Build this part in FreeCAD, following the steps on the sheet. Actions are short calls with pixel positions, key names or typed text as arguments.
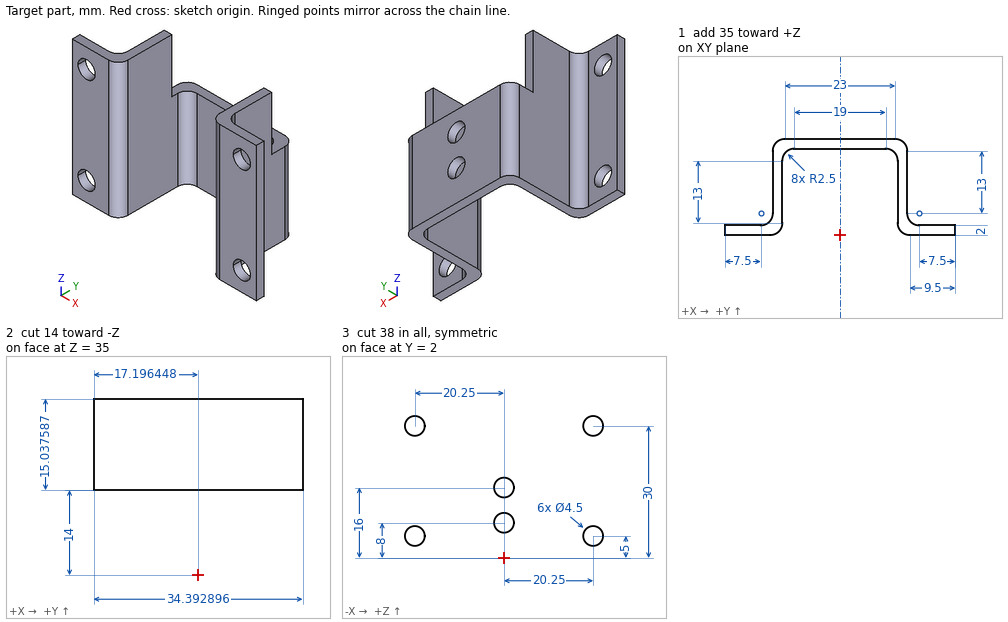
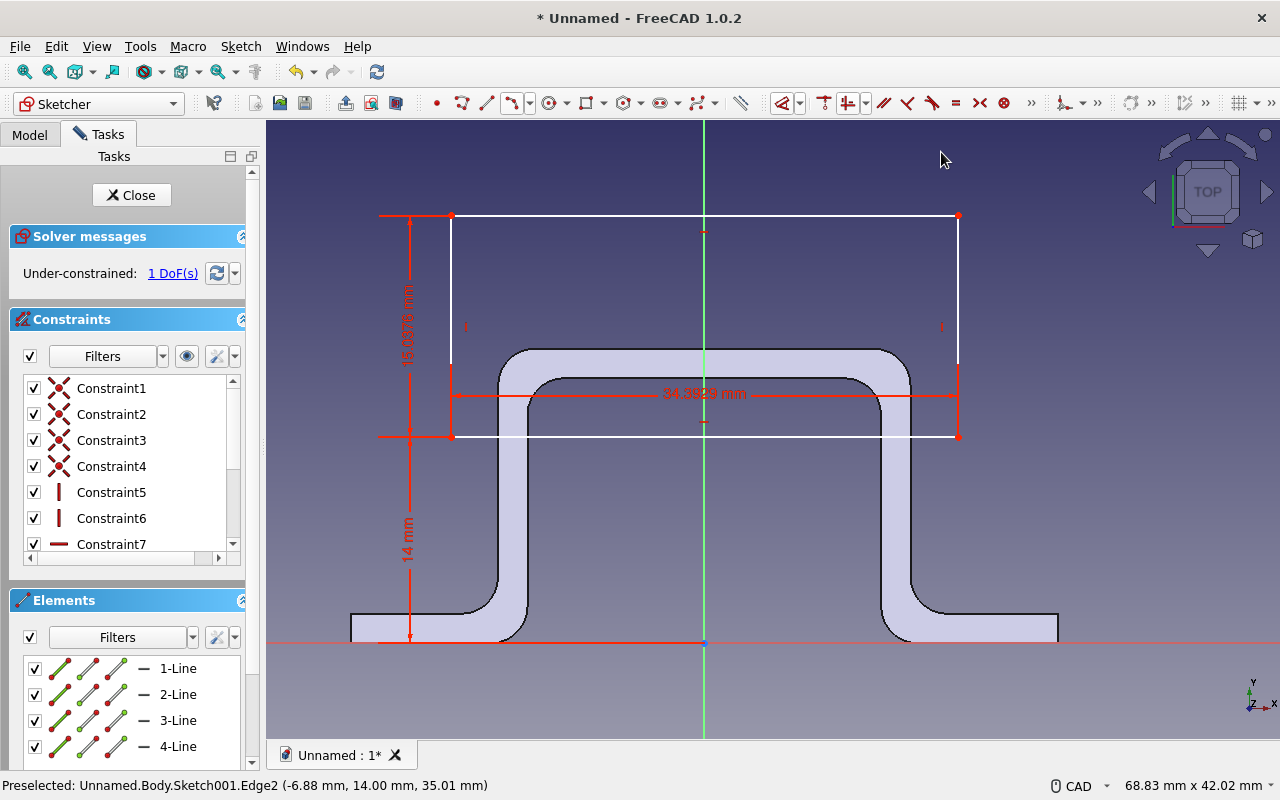
click(451, 216)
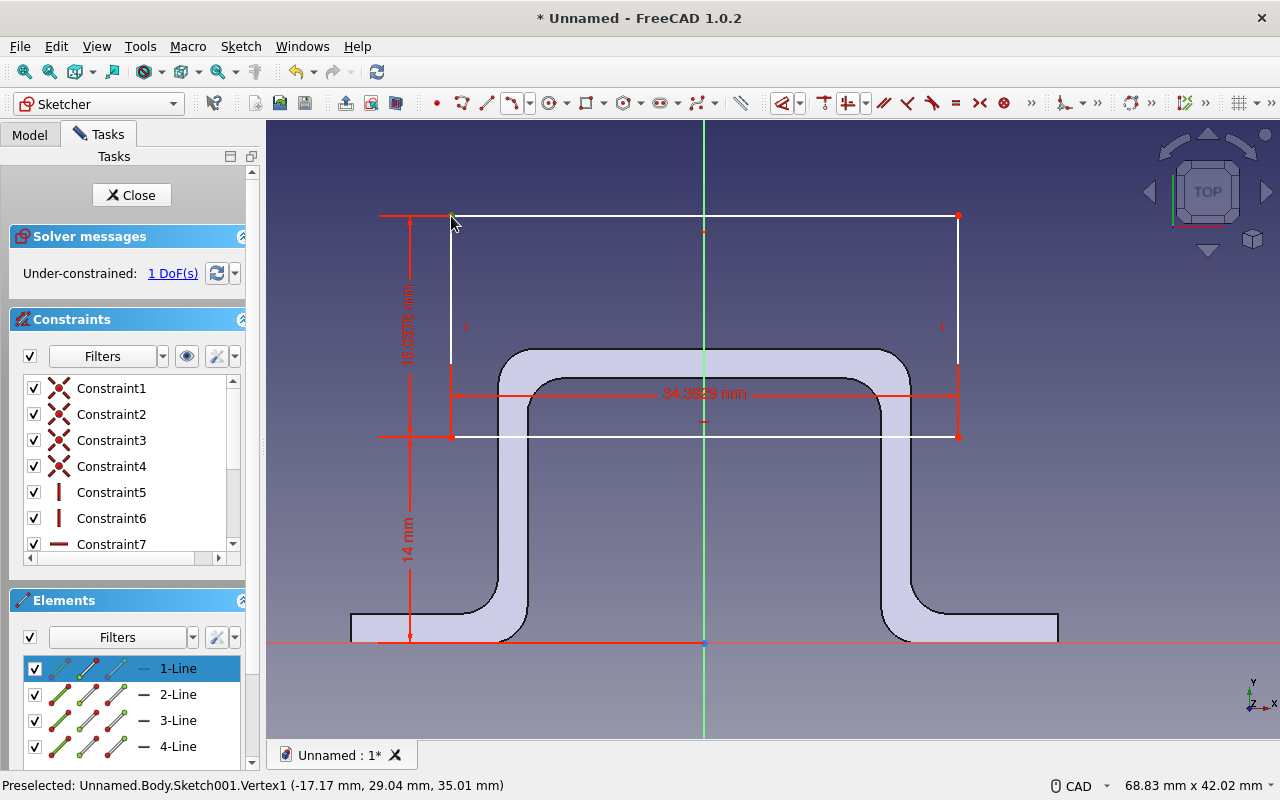
click(800, 104)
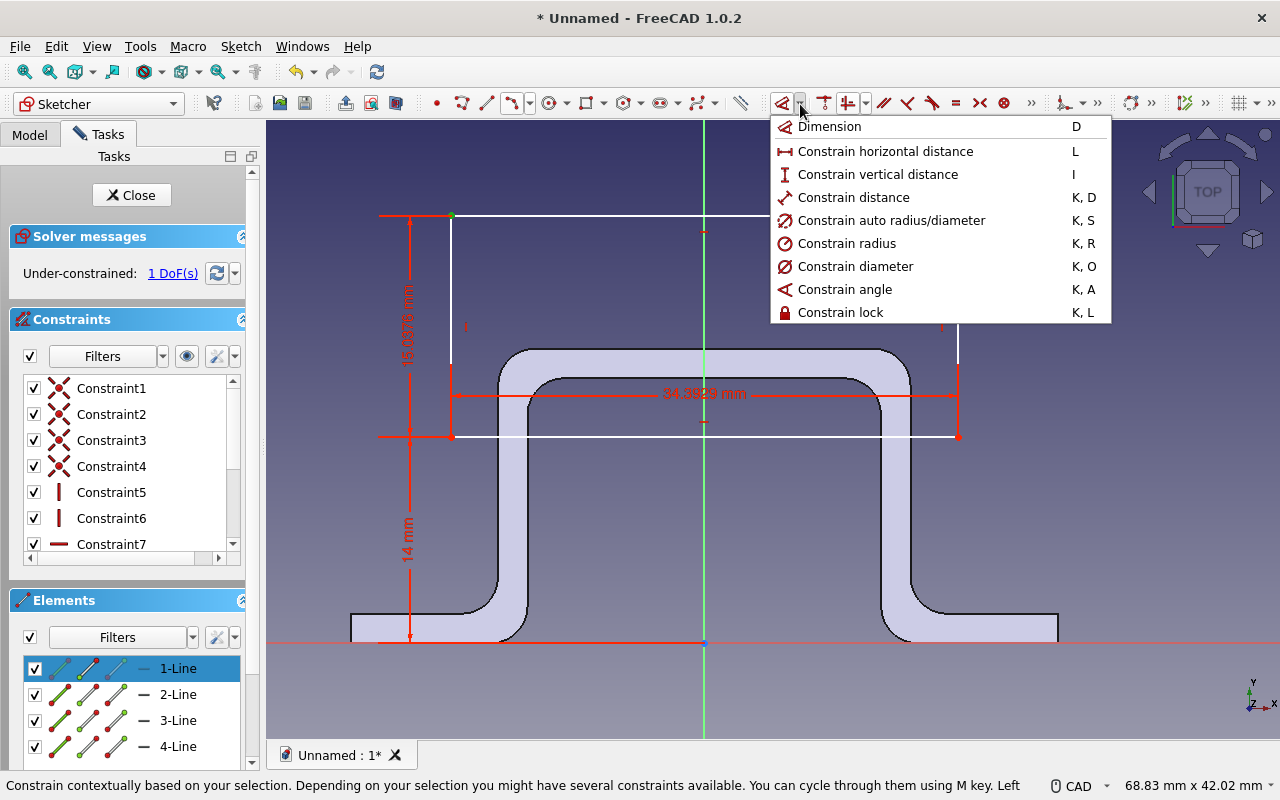
click(941, 152)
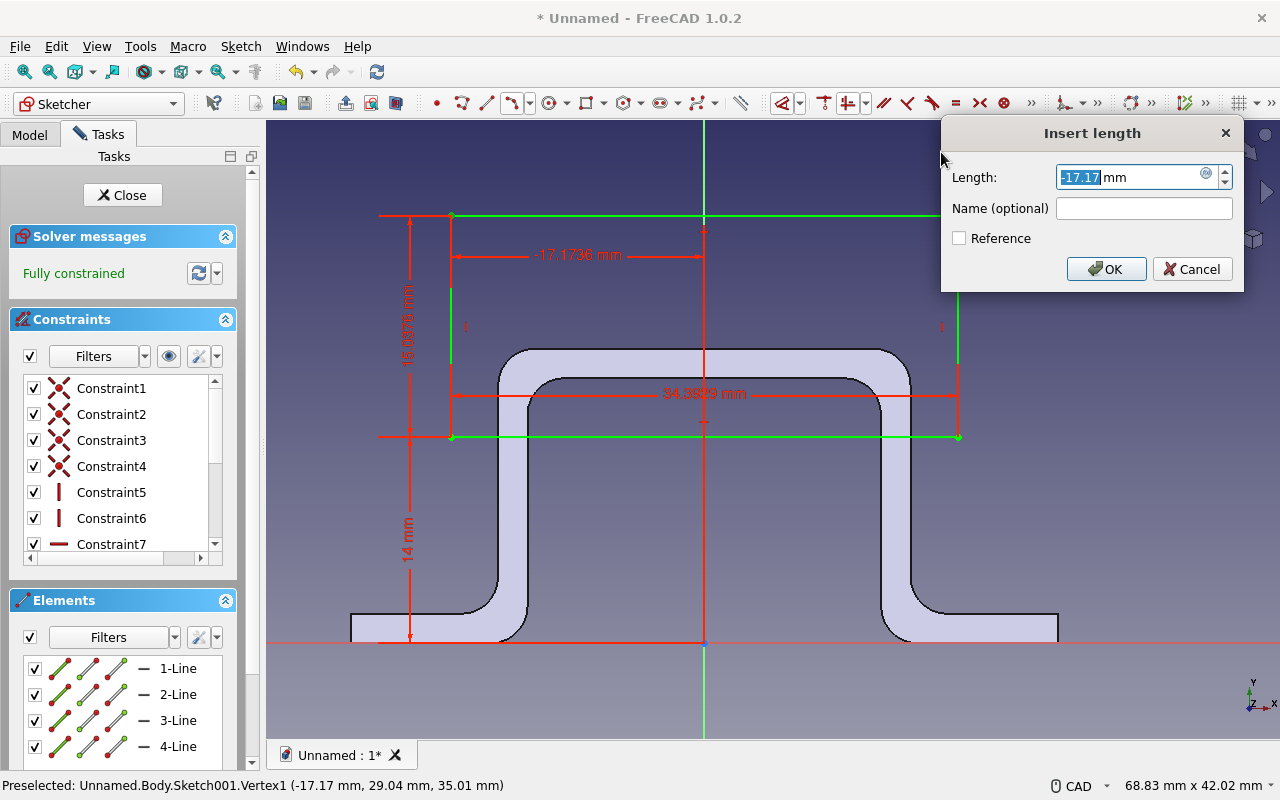
text(-17.196448)
key(Return)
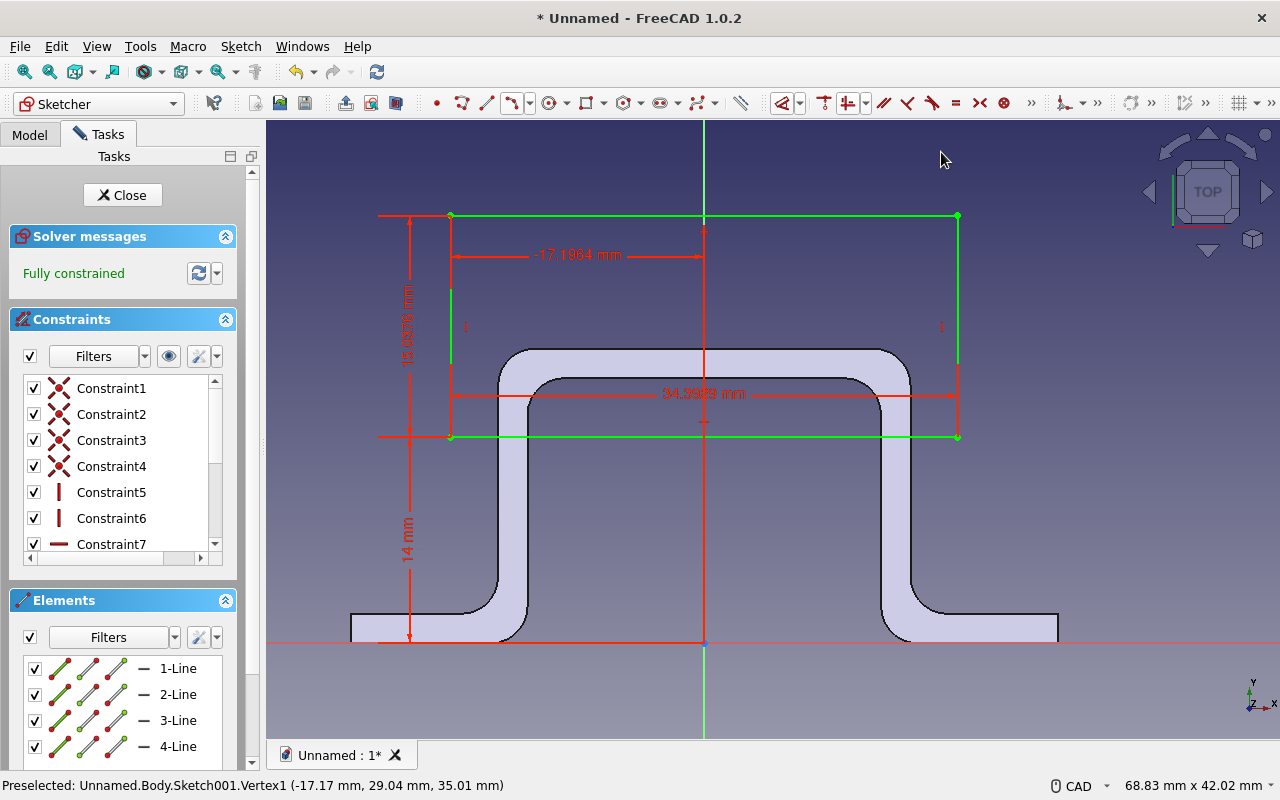
click(123, 195)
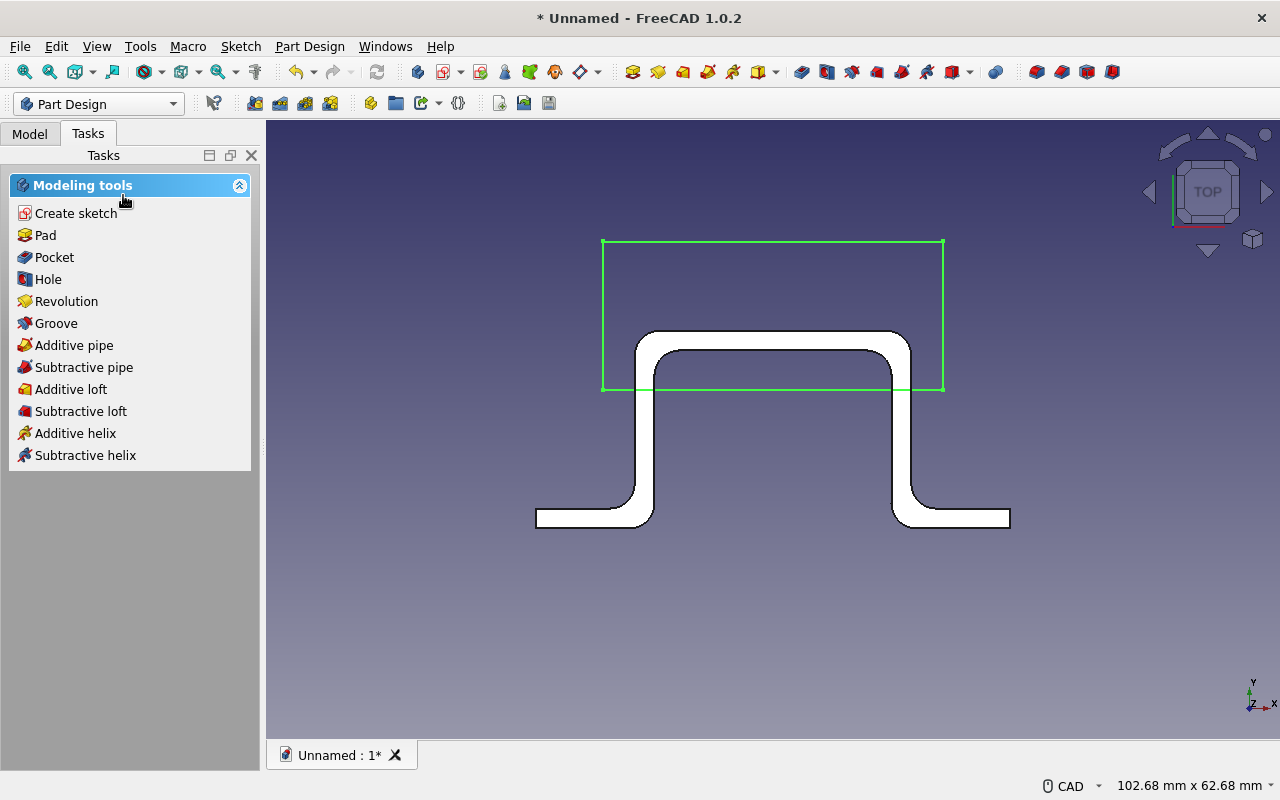
click(802, 72)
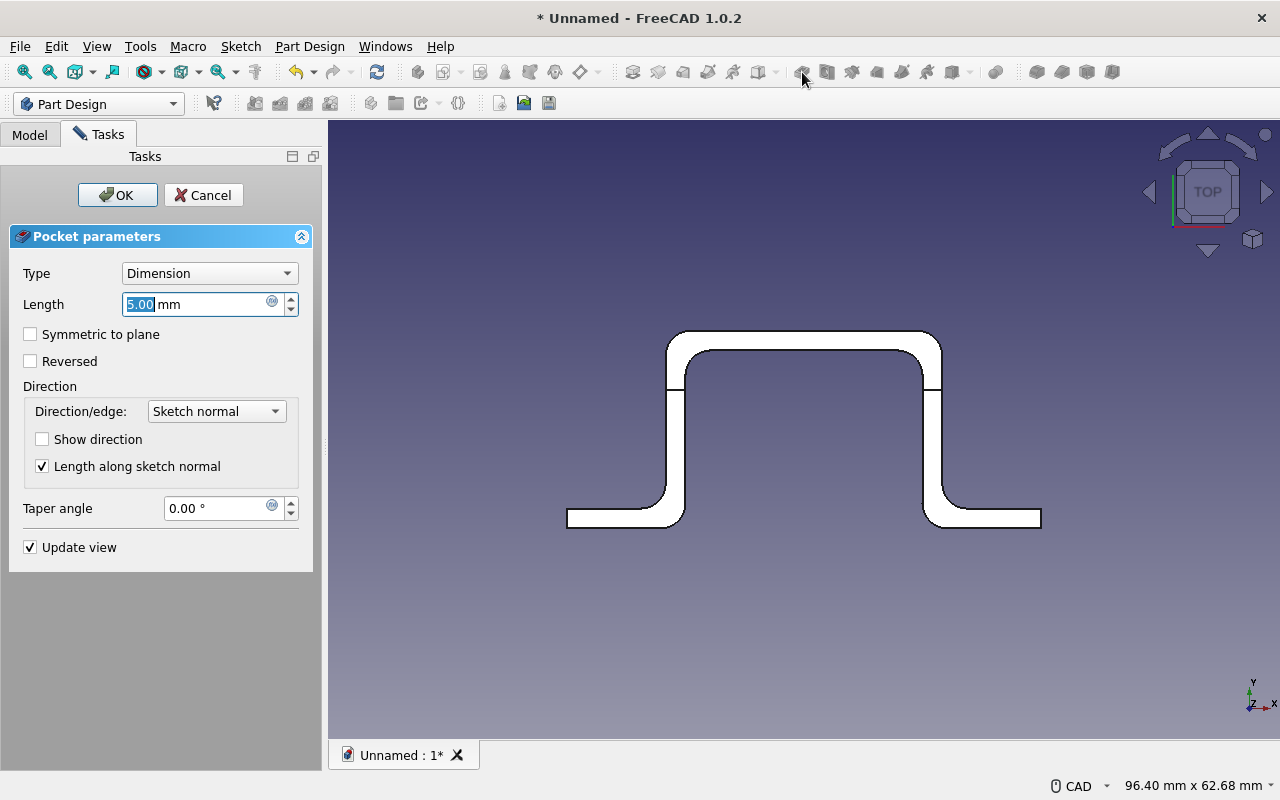
text(14)
key(Tab)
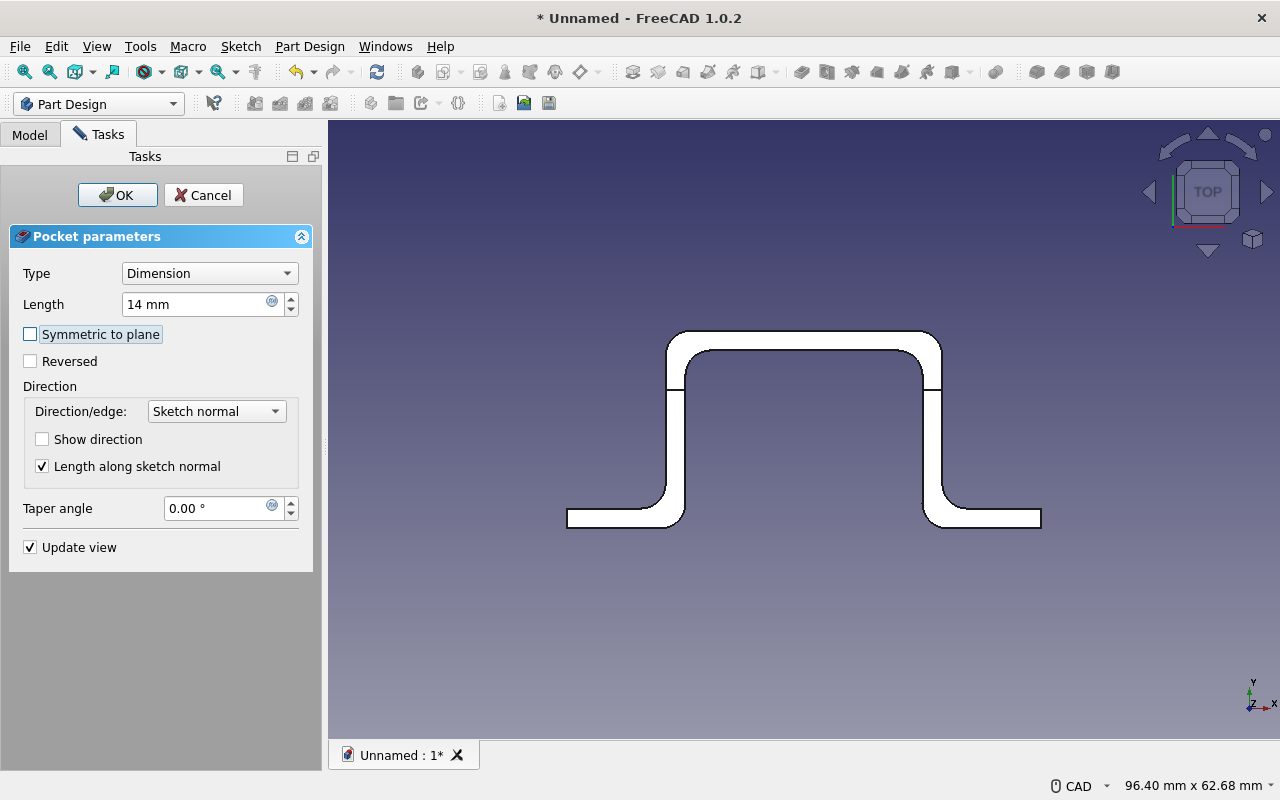
click(118, 195)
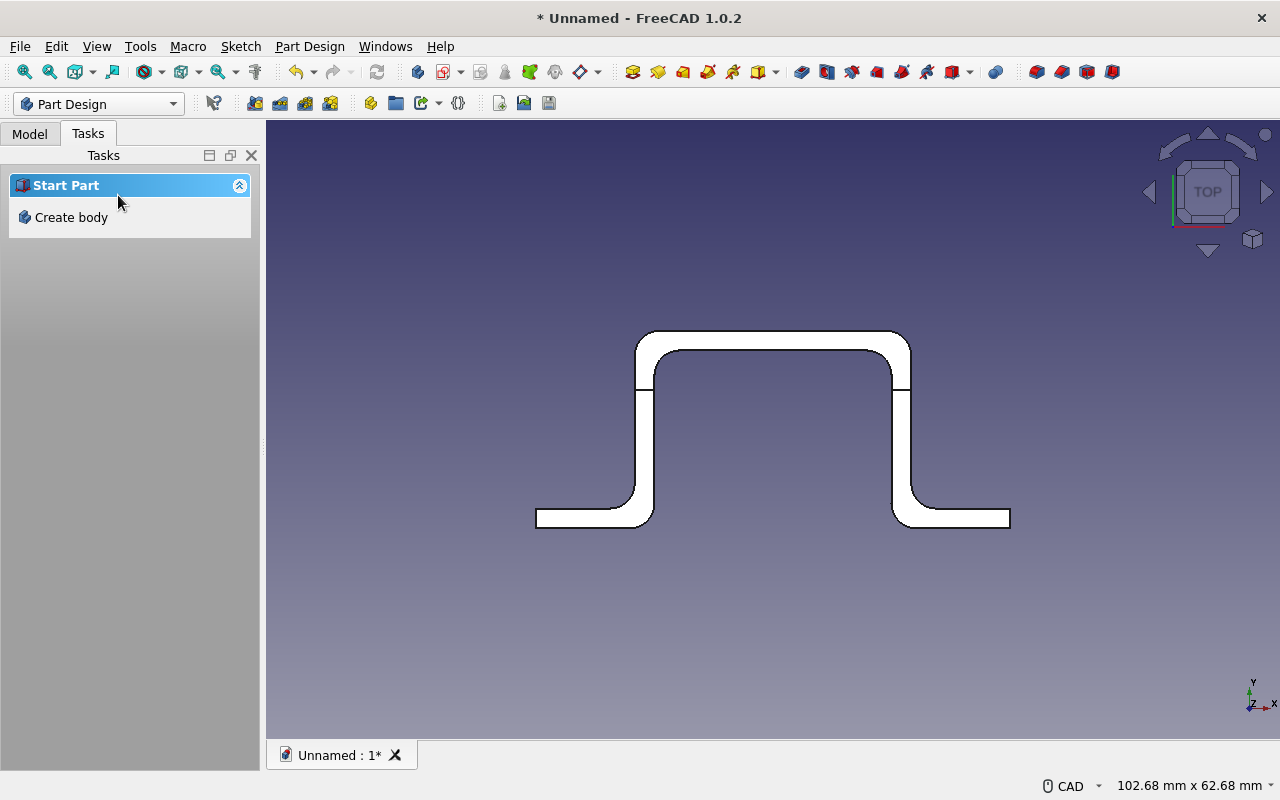
key(4)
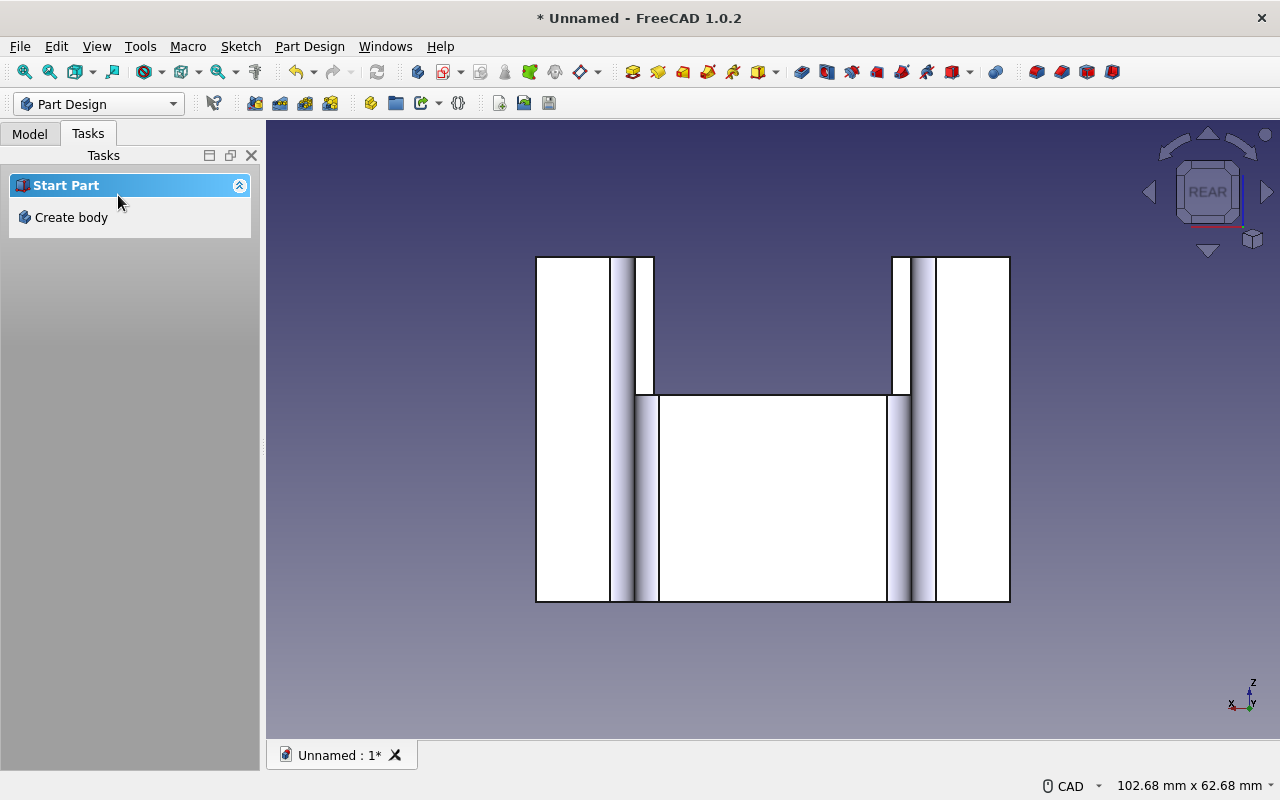
click(573, 330)